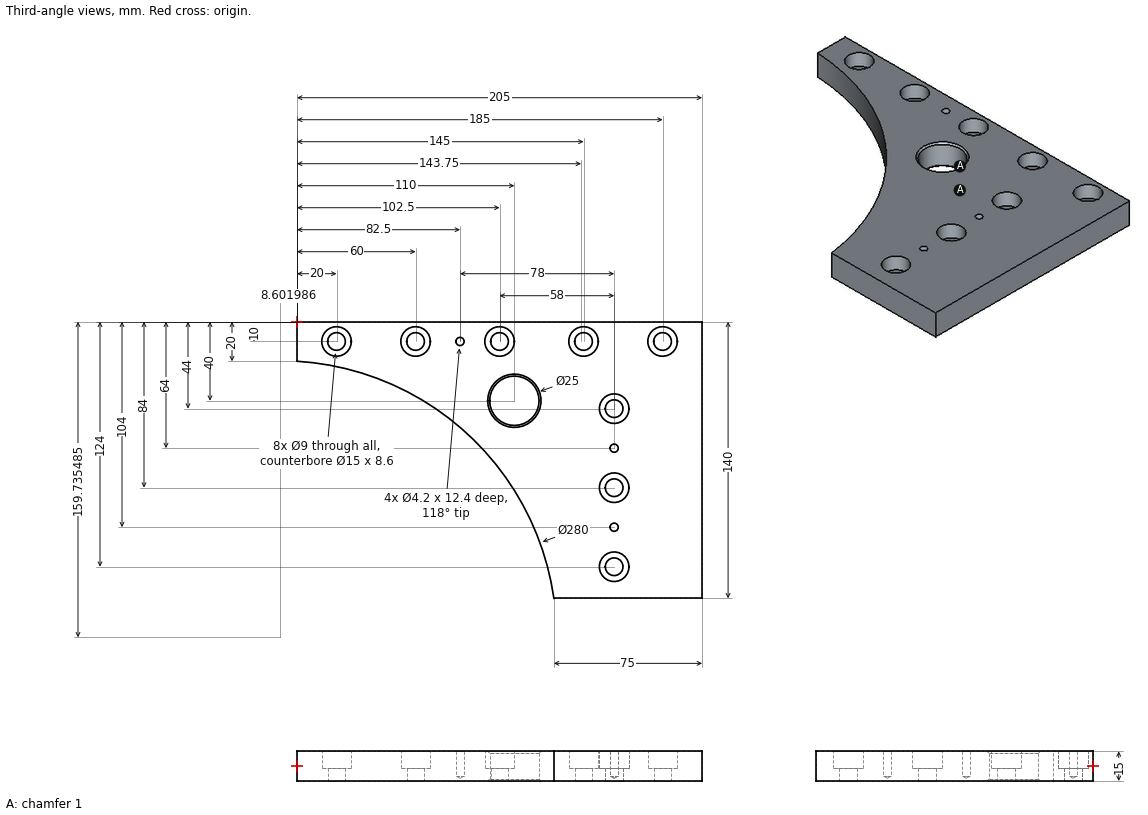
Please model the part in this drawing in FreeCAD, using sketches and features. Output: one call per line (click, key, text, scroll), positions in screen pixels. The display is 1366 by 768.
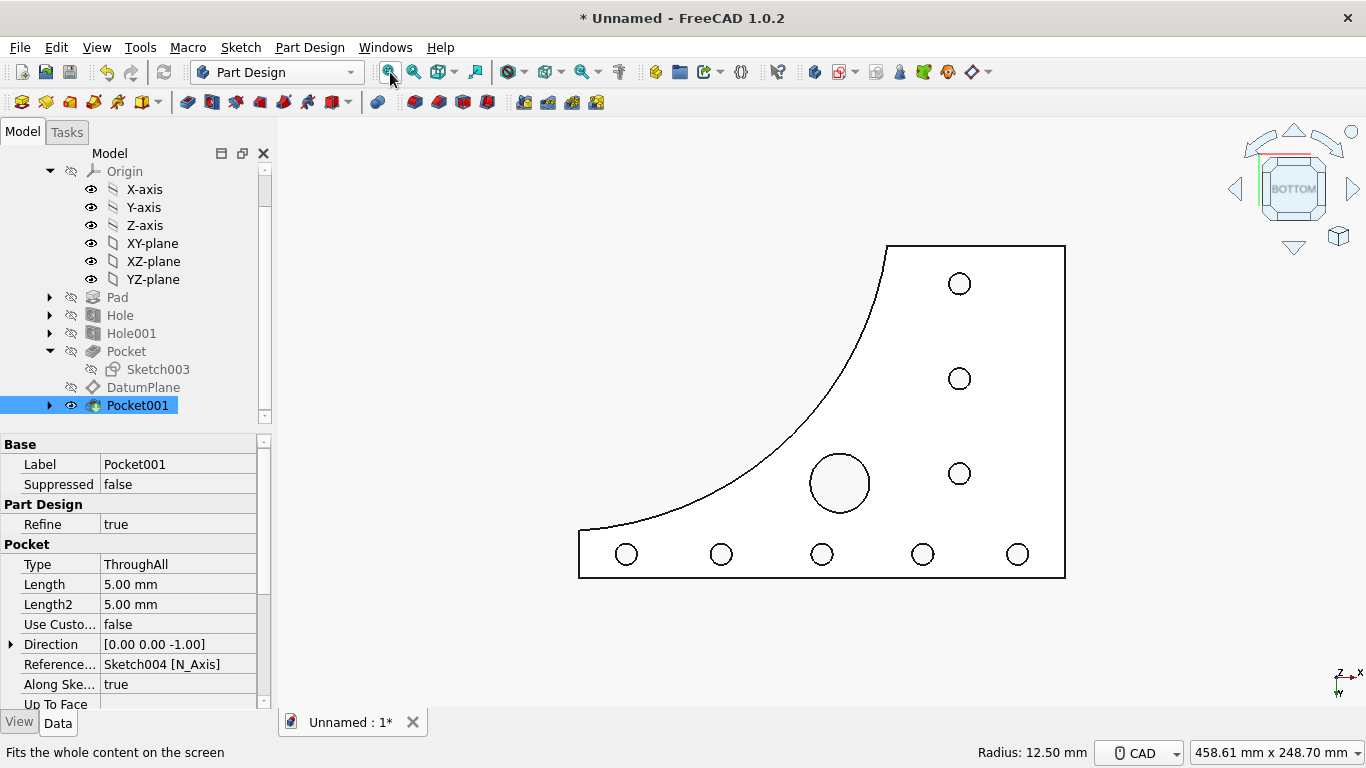
click(810, 482, ctrl)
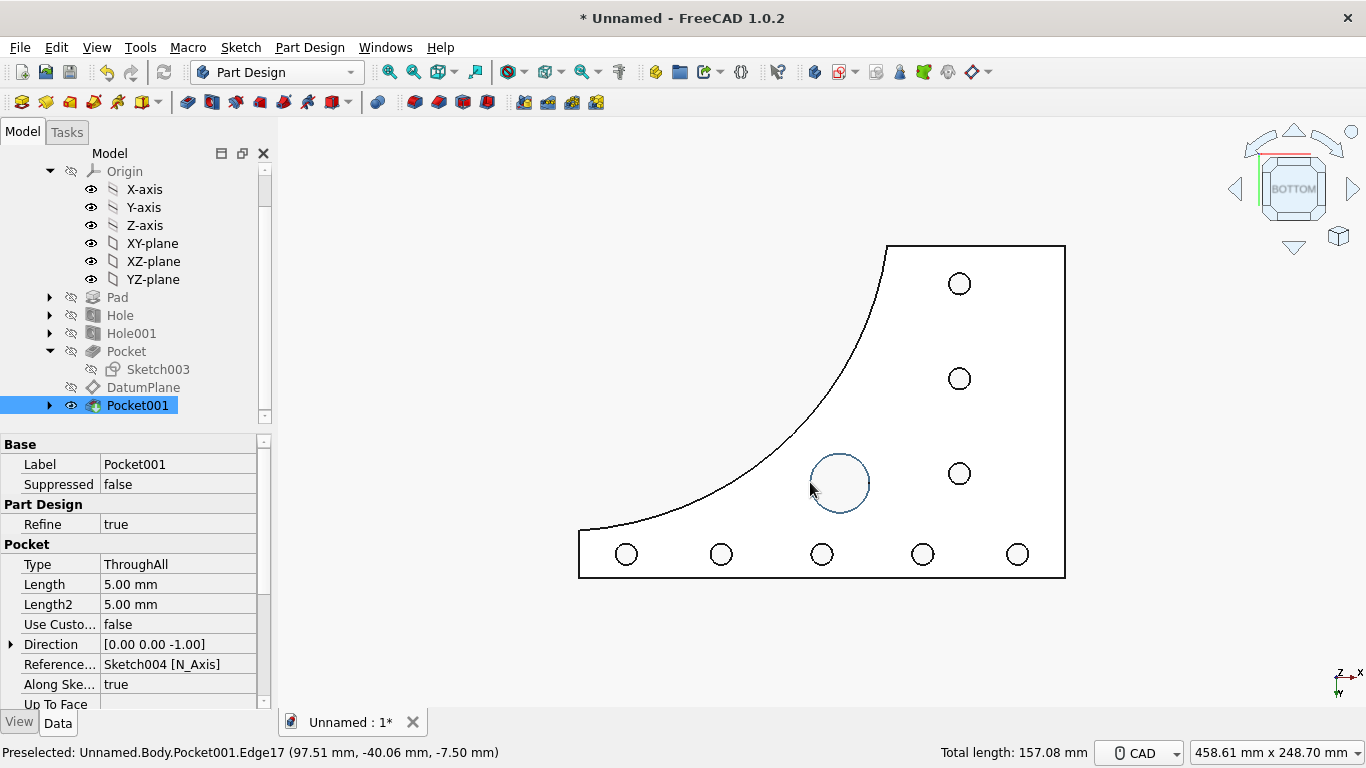
click(440, 102)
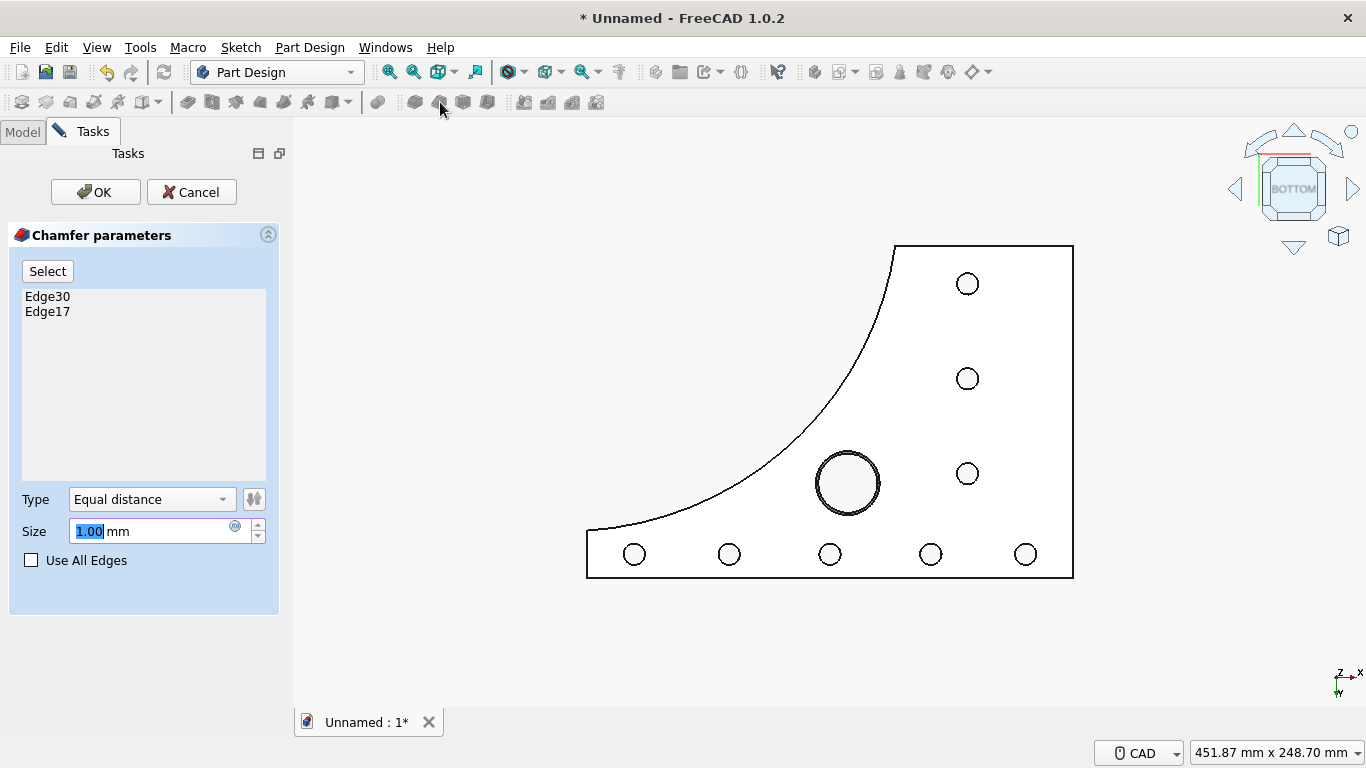
text(1)
key(Tab)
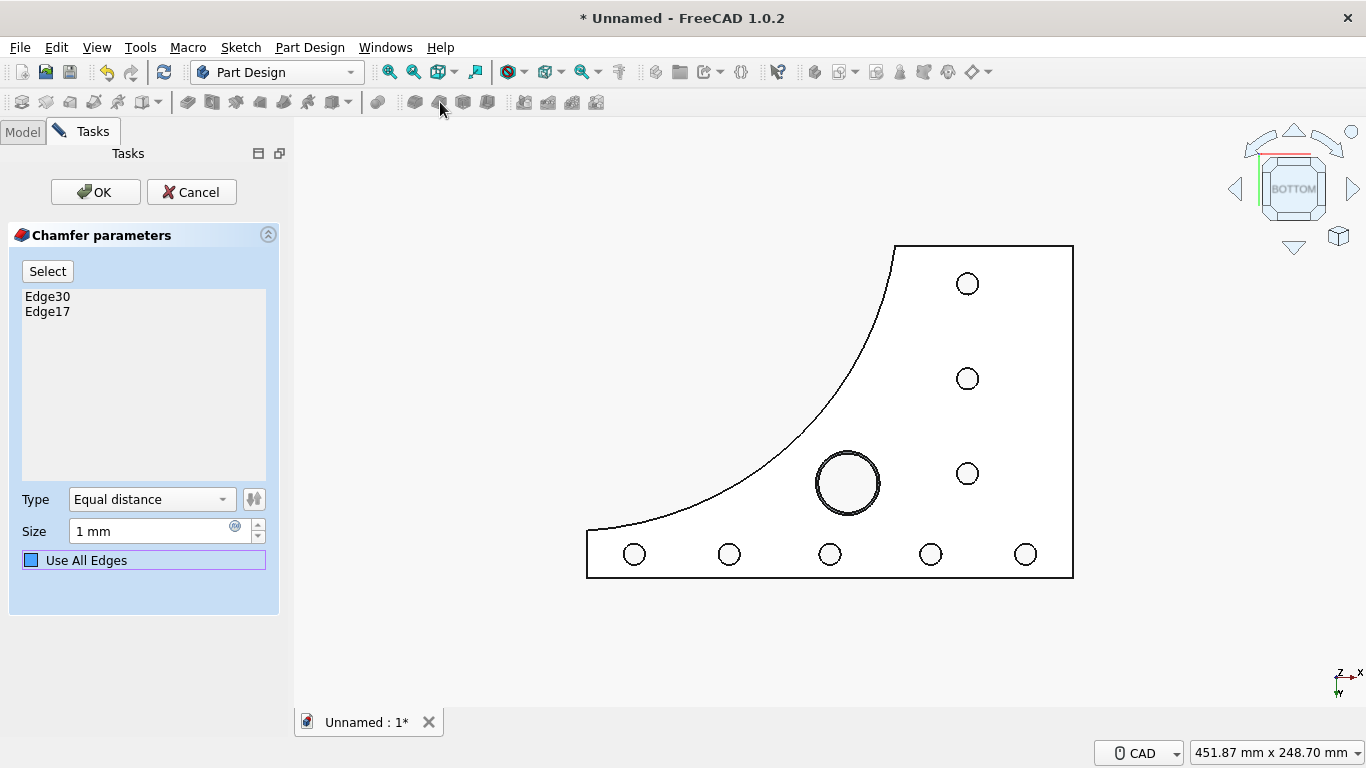
click(96, 192)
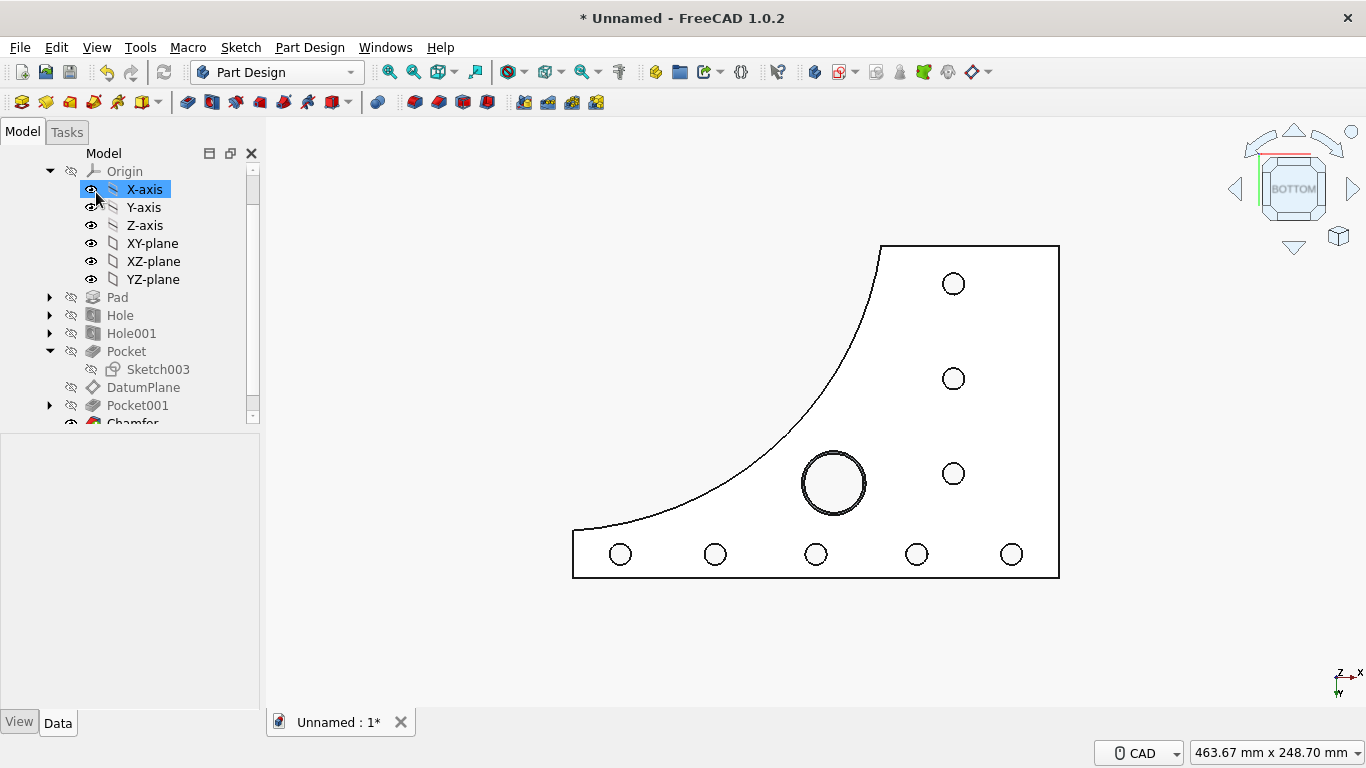
key(0)